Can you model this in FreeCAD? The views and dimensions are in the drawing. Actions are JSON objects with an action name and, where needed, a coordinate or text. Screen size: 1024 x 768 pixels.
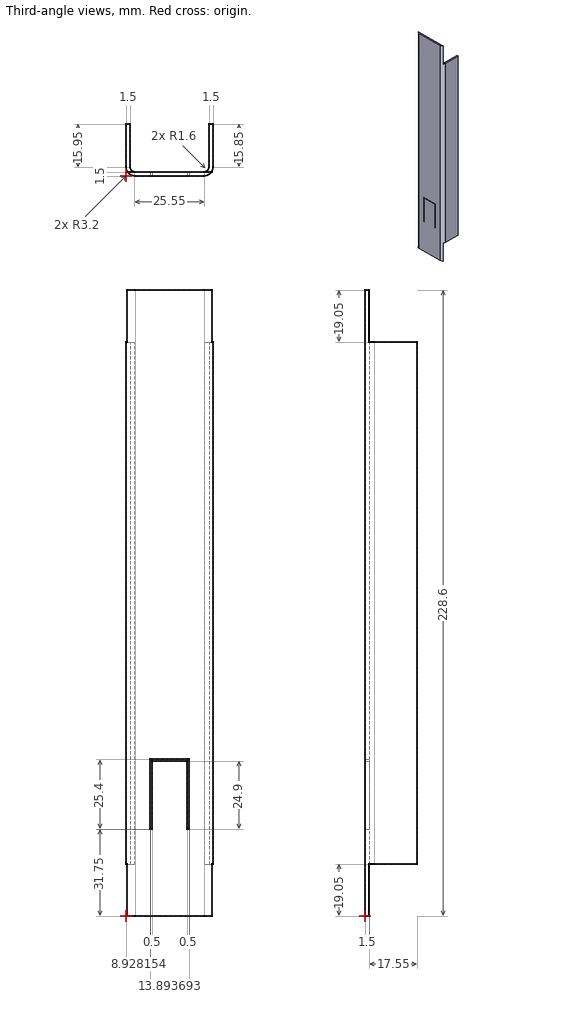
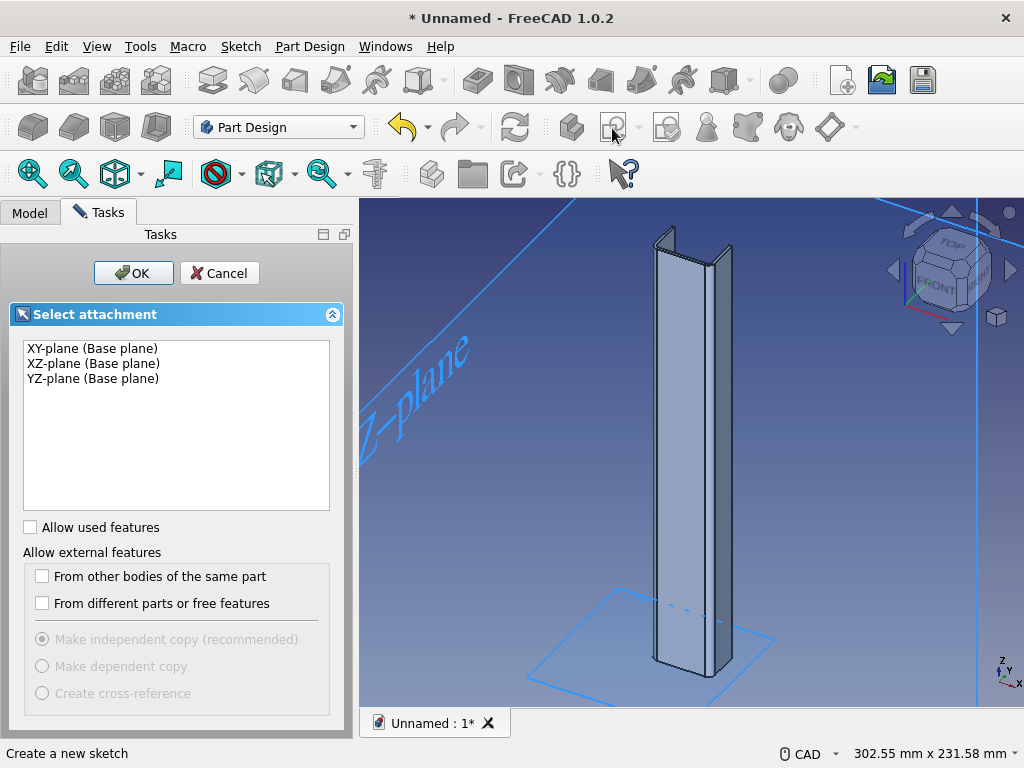
{"action": "left_click", "coordinate": [84, 378]}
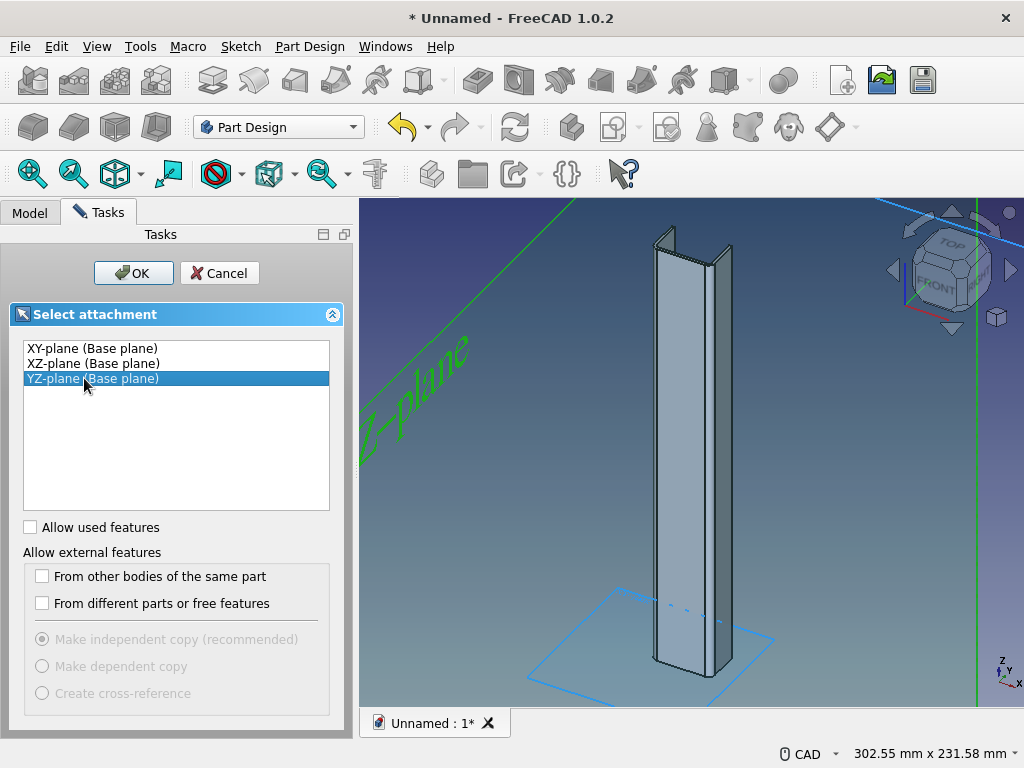
{"action": "left_click", "coordinate": [134, 273]}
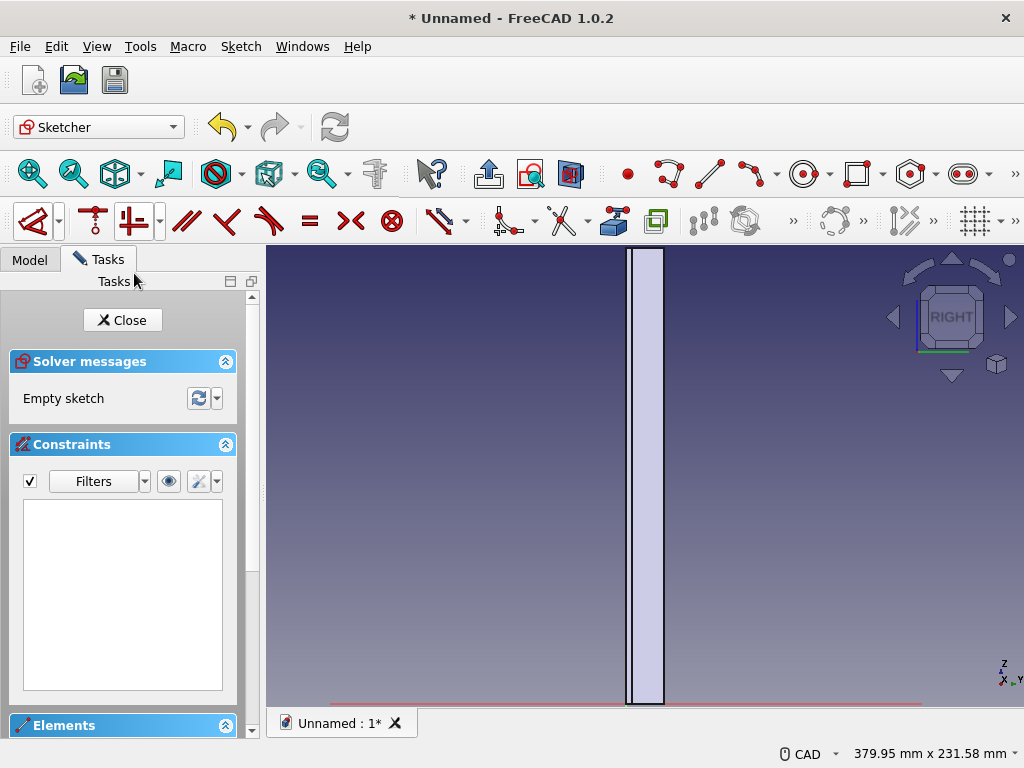
{"action": "left_click", "coordinate": [571, 174]}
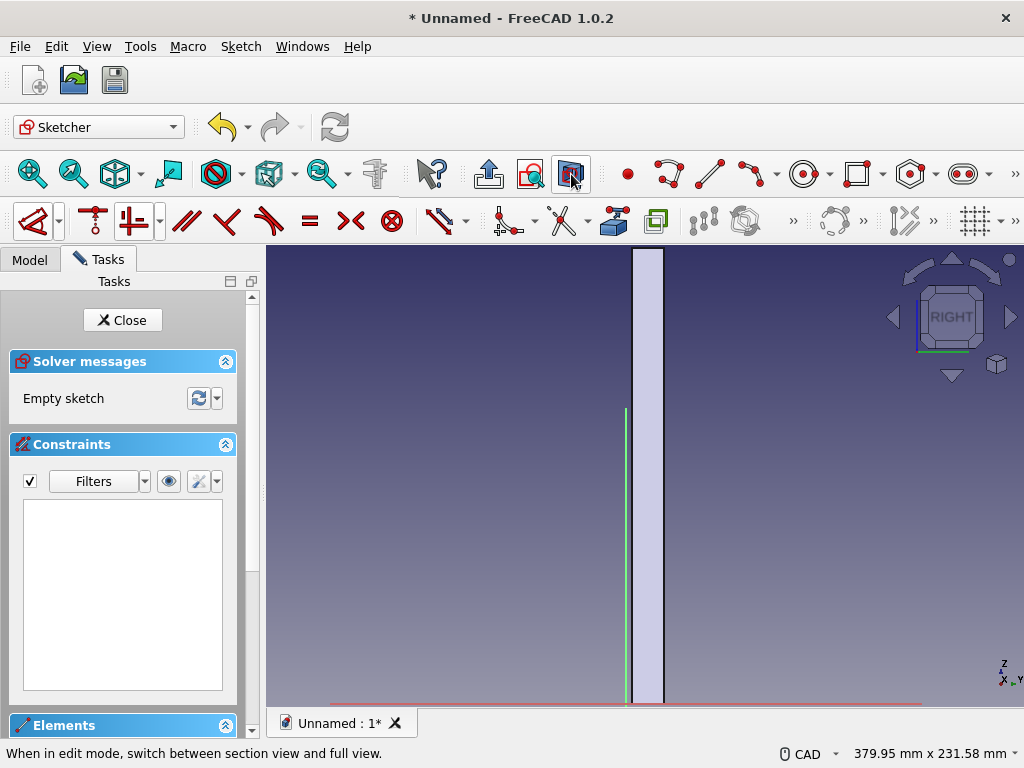
{"action": "scroll", "coordinate": [437, 476], "scroll_direction": "down", "scroll_amount": 2}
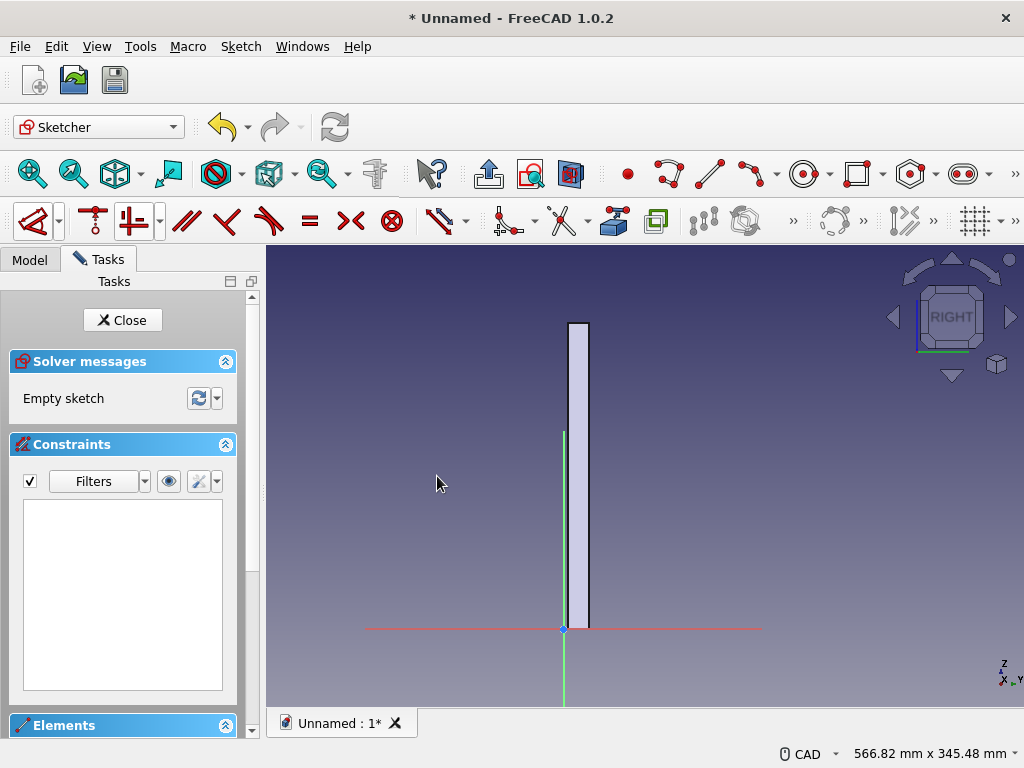
{"action": "left_click", "coordinate": [856, 174]}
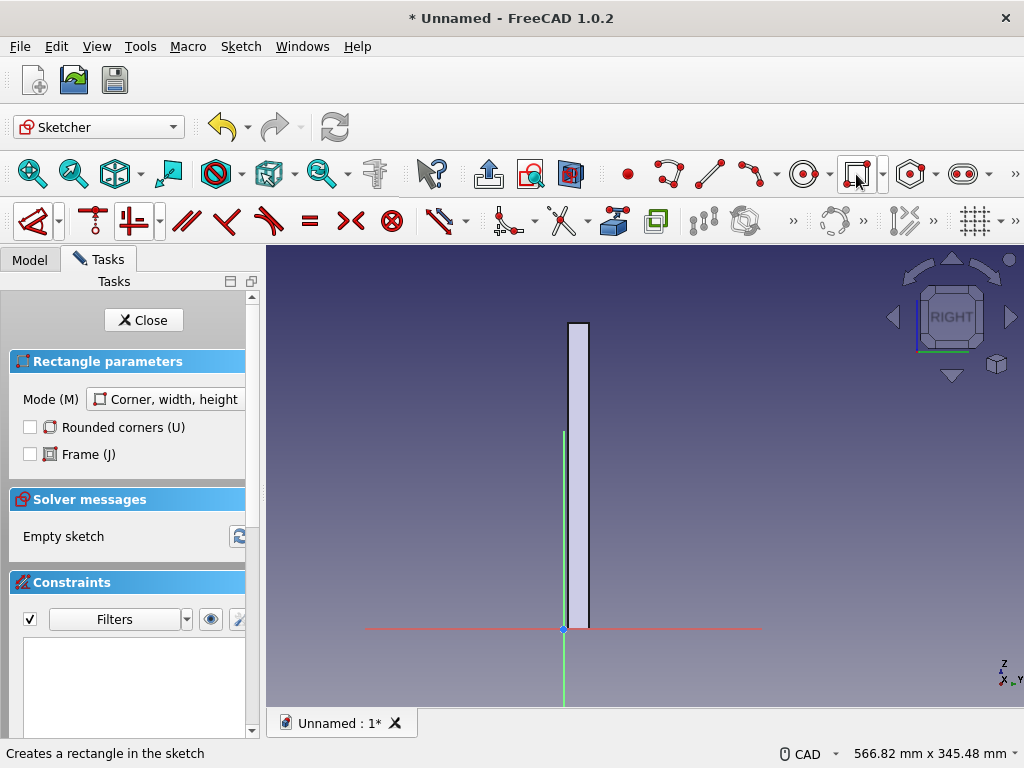
{"action": "scroll", "coordinate": [566, 604], "scroll_direction": "up", "scroll_amount": 11}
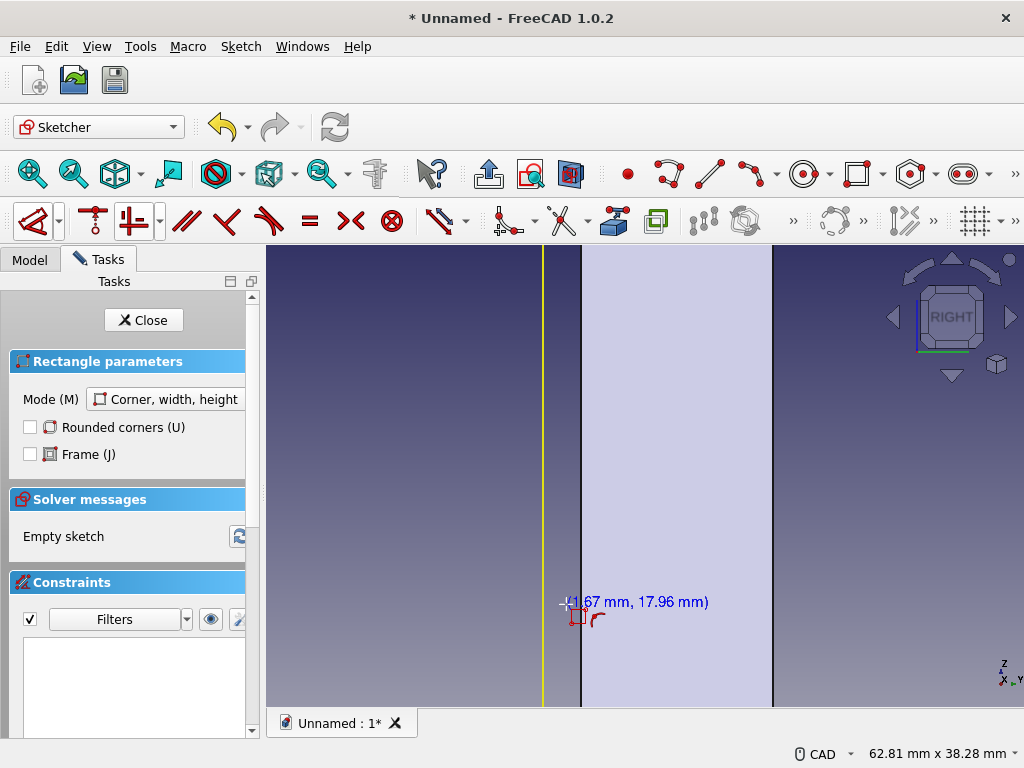
{"action": "left_click", "coordinate": [561, 594]}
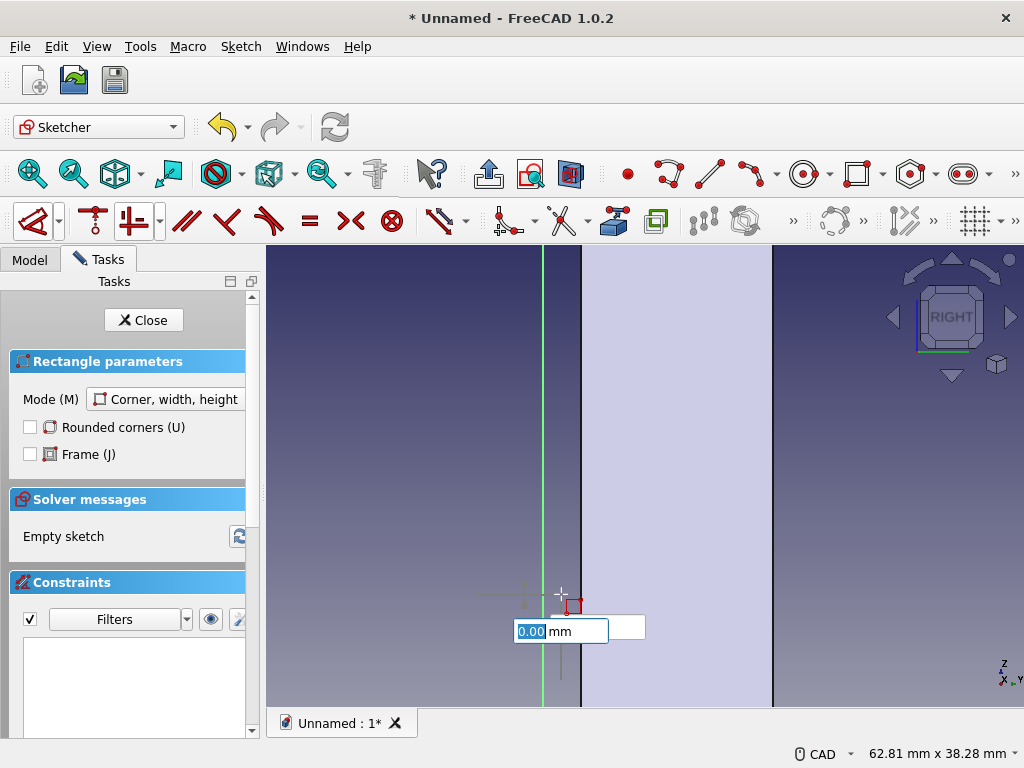
{"action": "scroll", "coordinate": [566, 605], "scroll_direction": "down", "scroll_amount": 11}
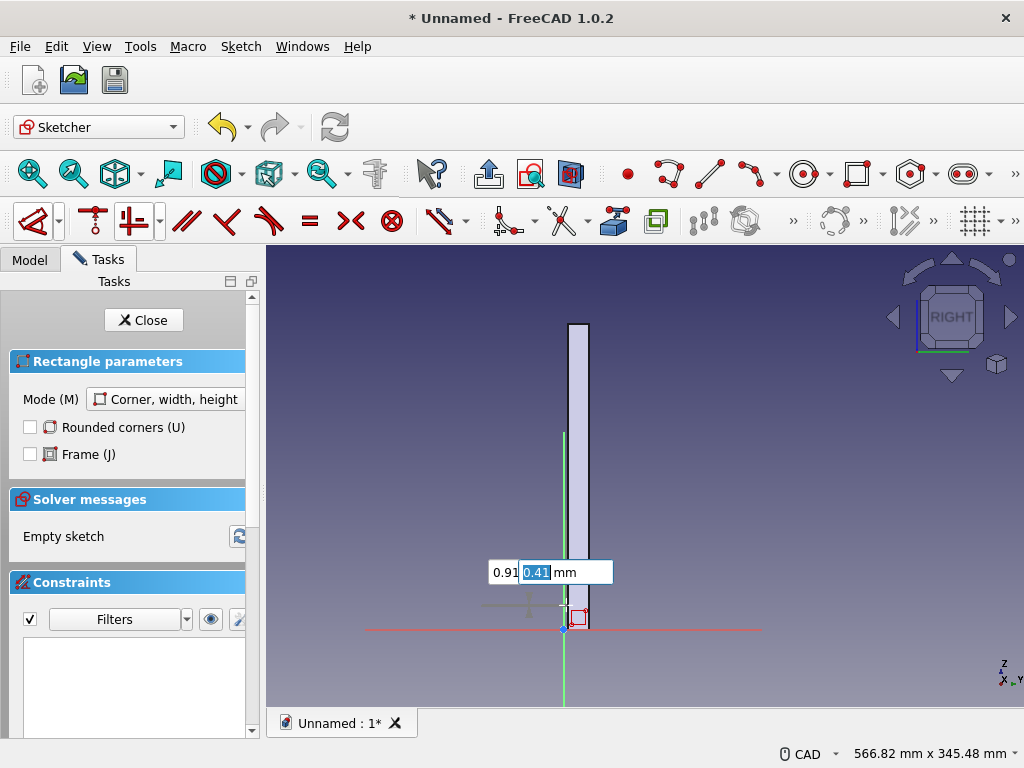
{"action": "left_click", "coordinate": [589, 630]}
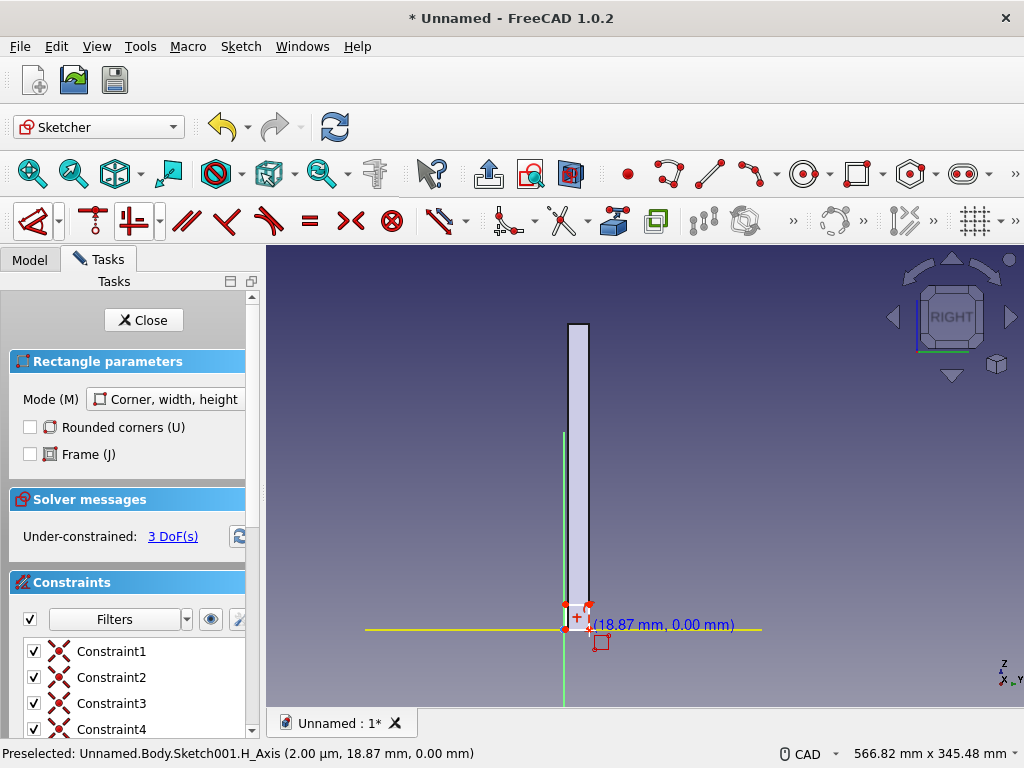
{"action": "scroll", "coordinate": [566, 324], "scroll_direction": "up", "scroll_amount": 11}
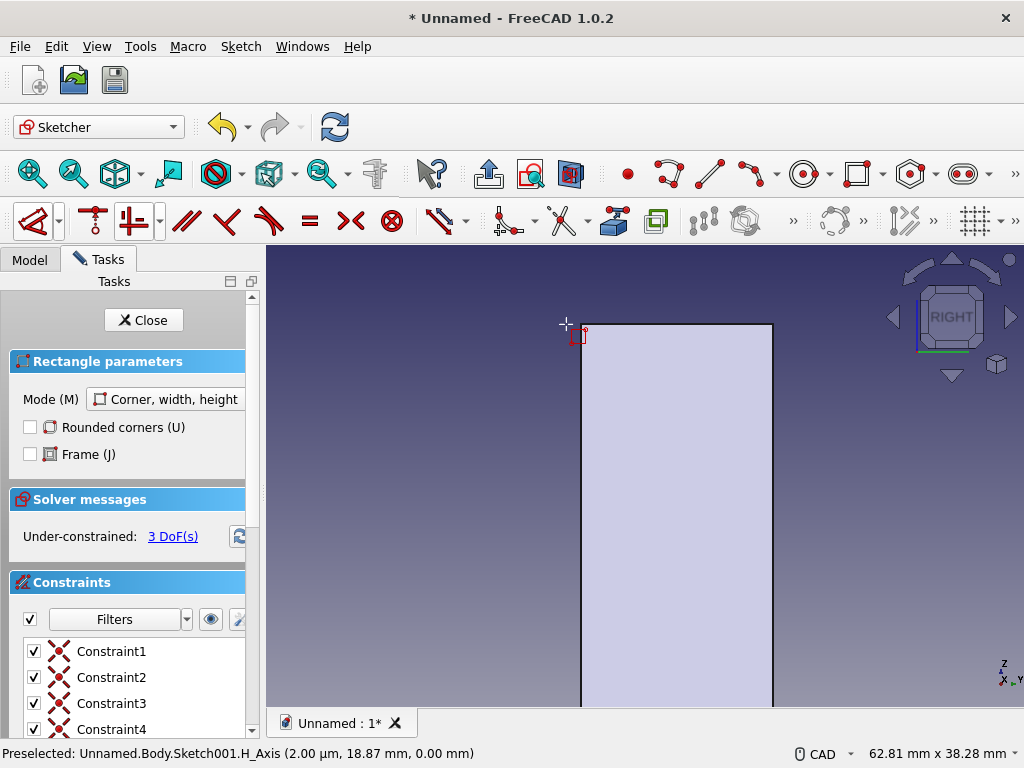
{"action": "left_click", "coordinate": [561, 324]}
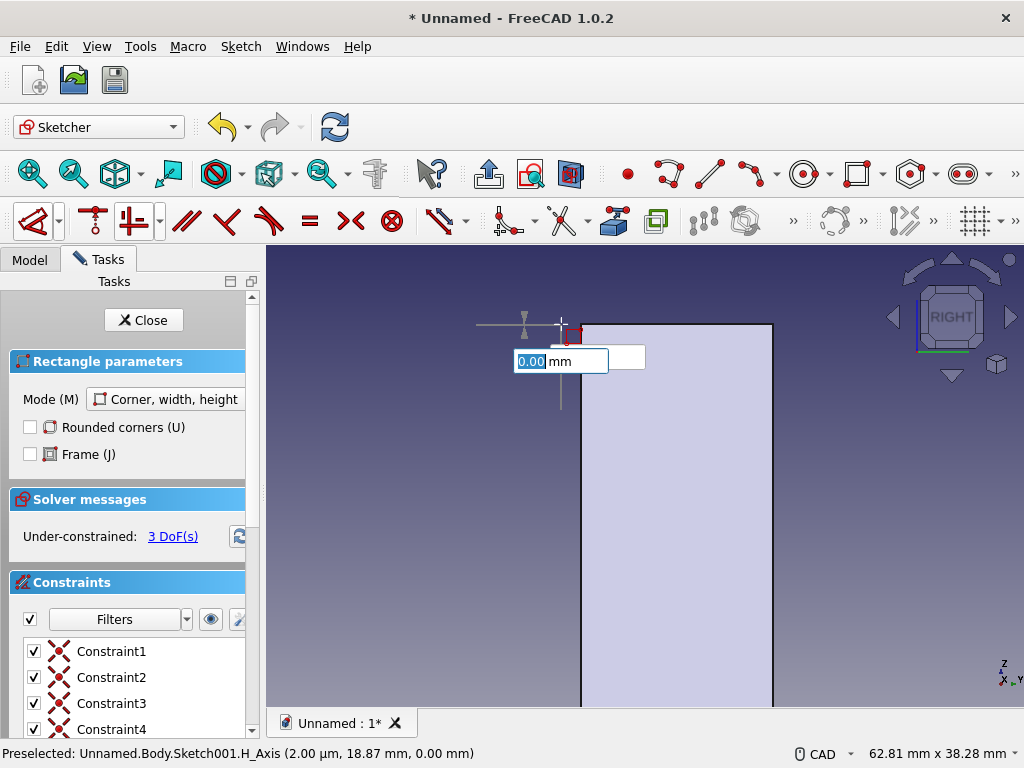
{"action": "scroll", "coordinate": [566, 323], "scroll_direction": "down", "scroll_amount": 11}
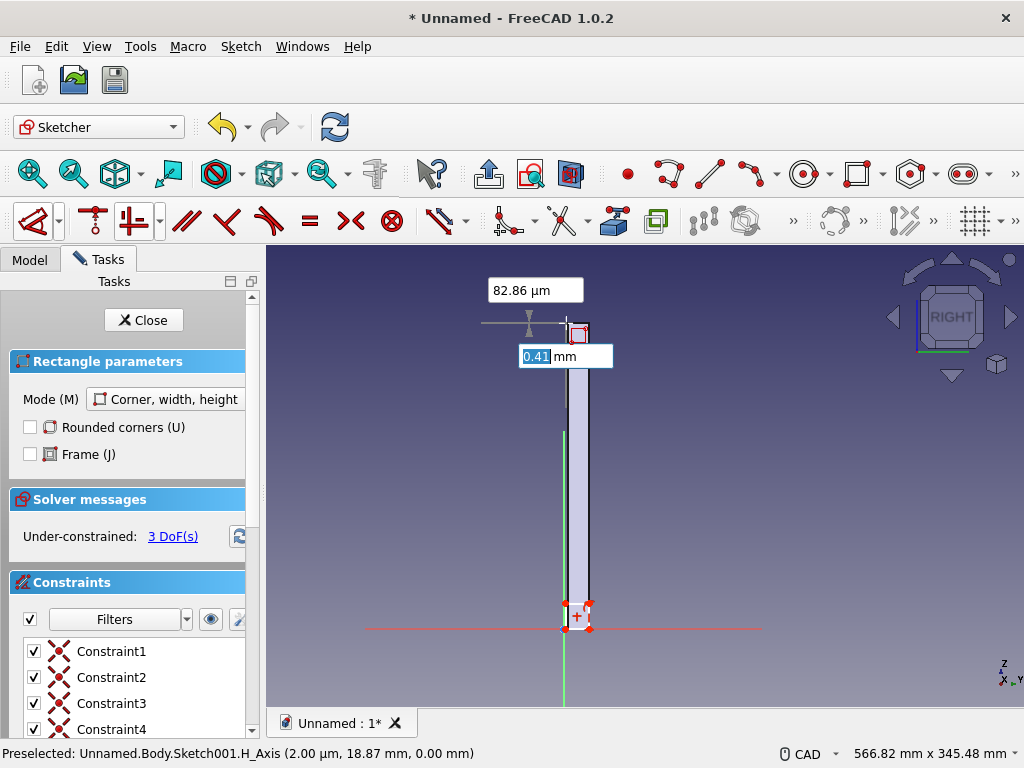
{"action": "left_click", "coordinate": [589, 349]}
{"action": "key", "text": "Escape"}